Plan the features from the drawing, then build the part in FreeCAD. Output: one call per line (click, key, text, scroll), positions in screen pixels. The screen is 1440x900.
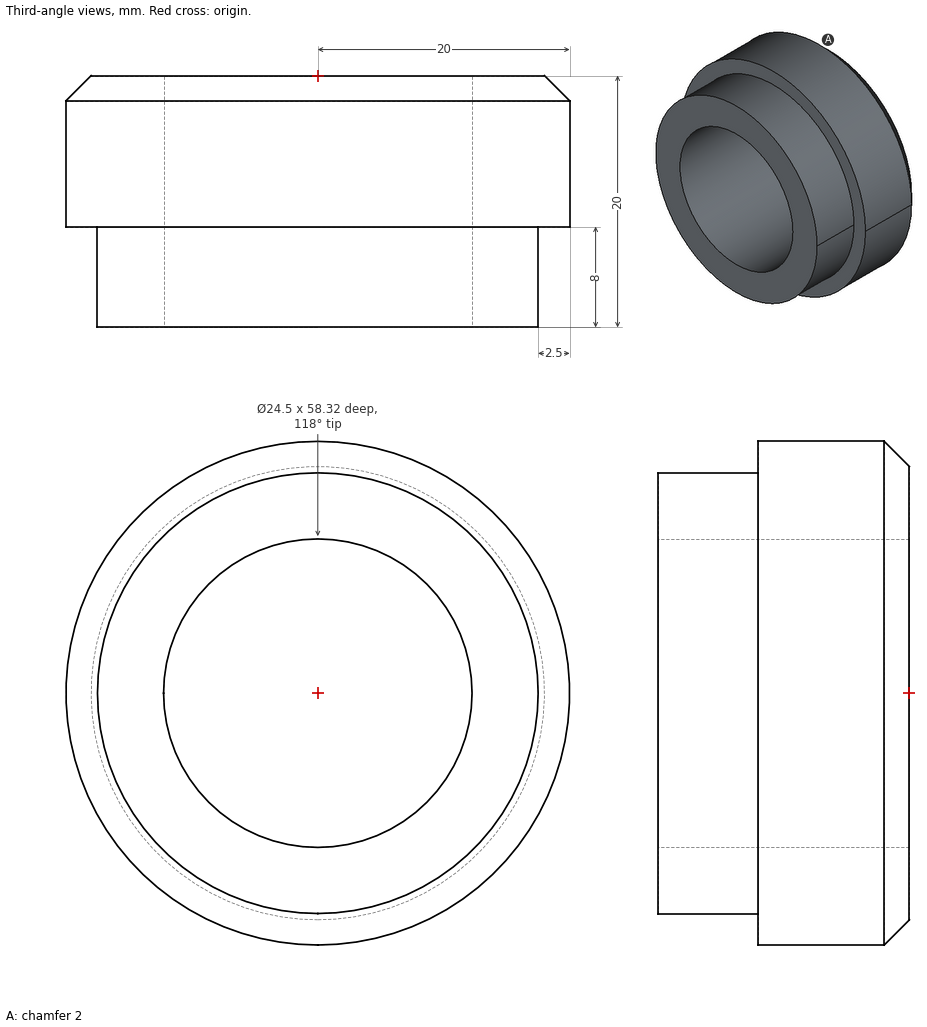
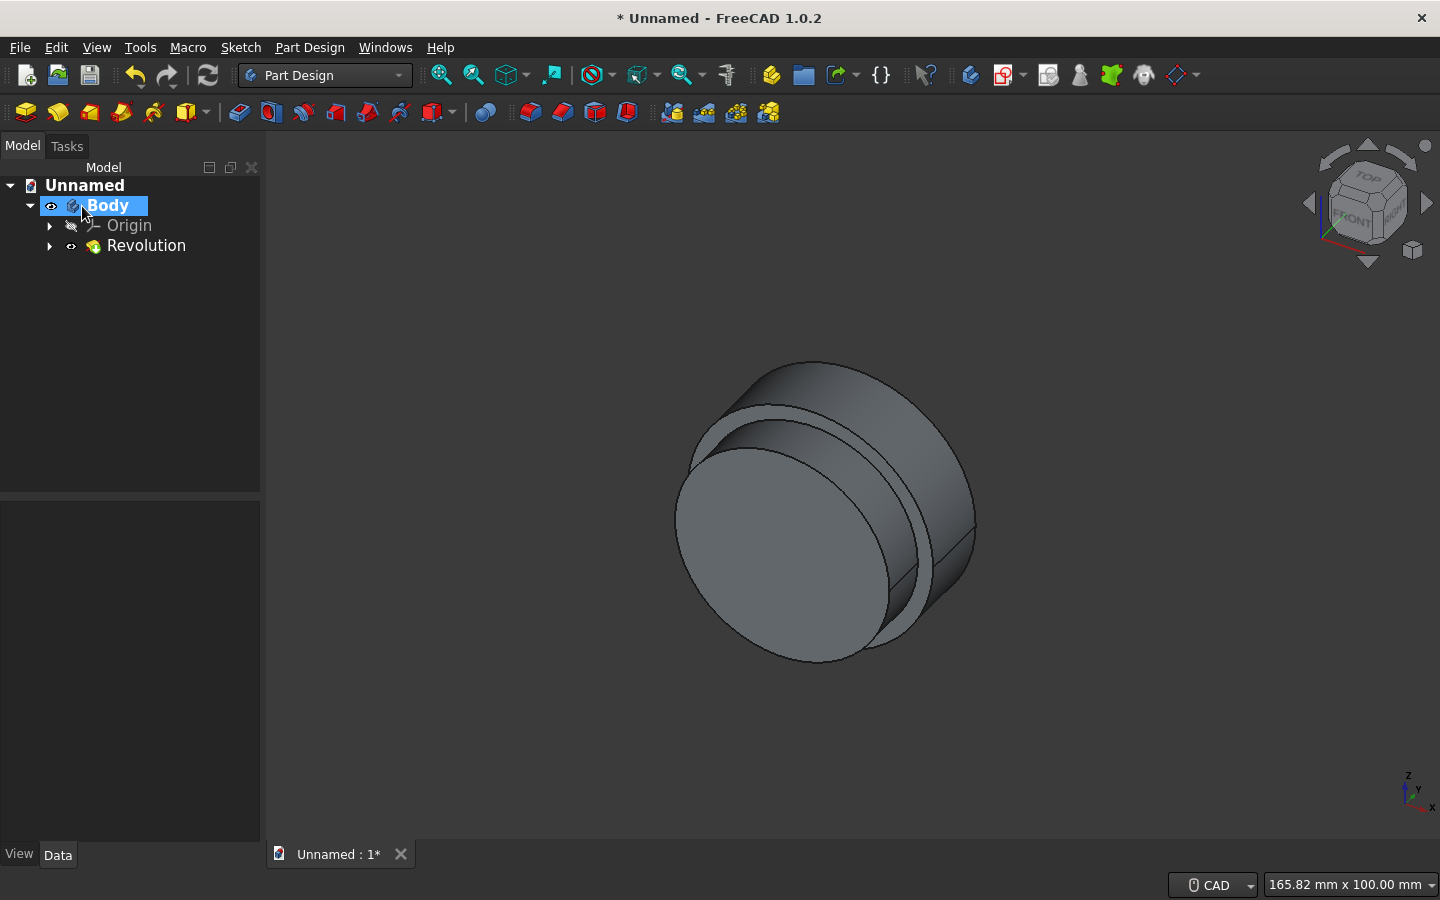
key(4)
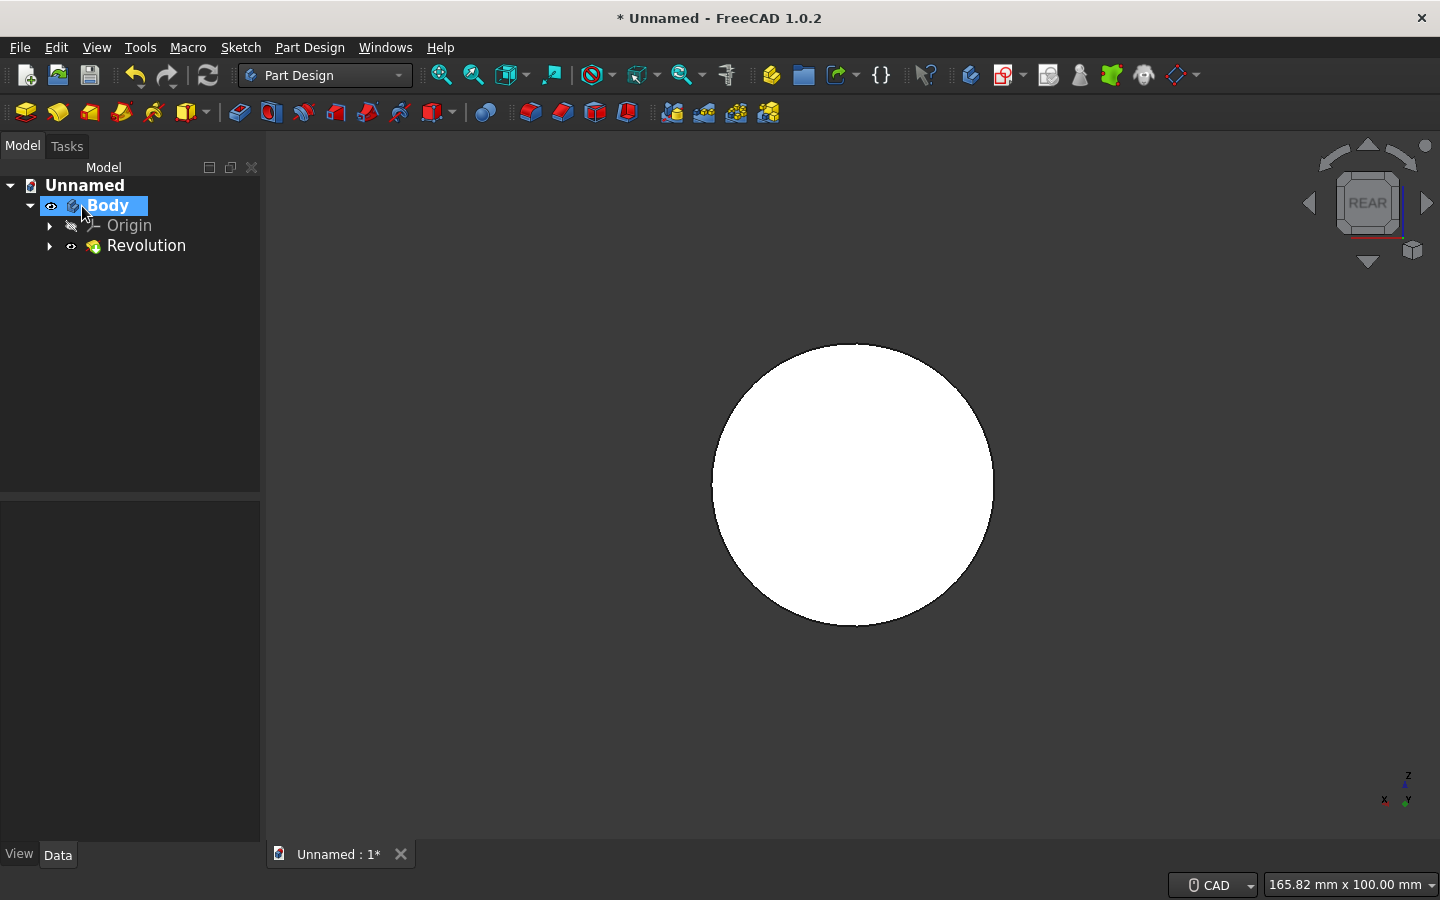
click(442, 76)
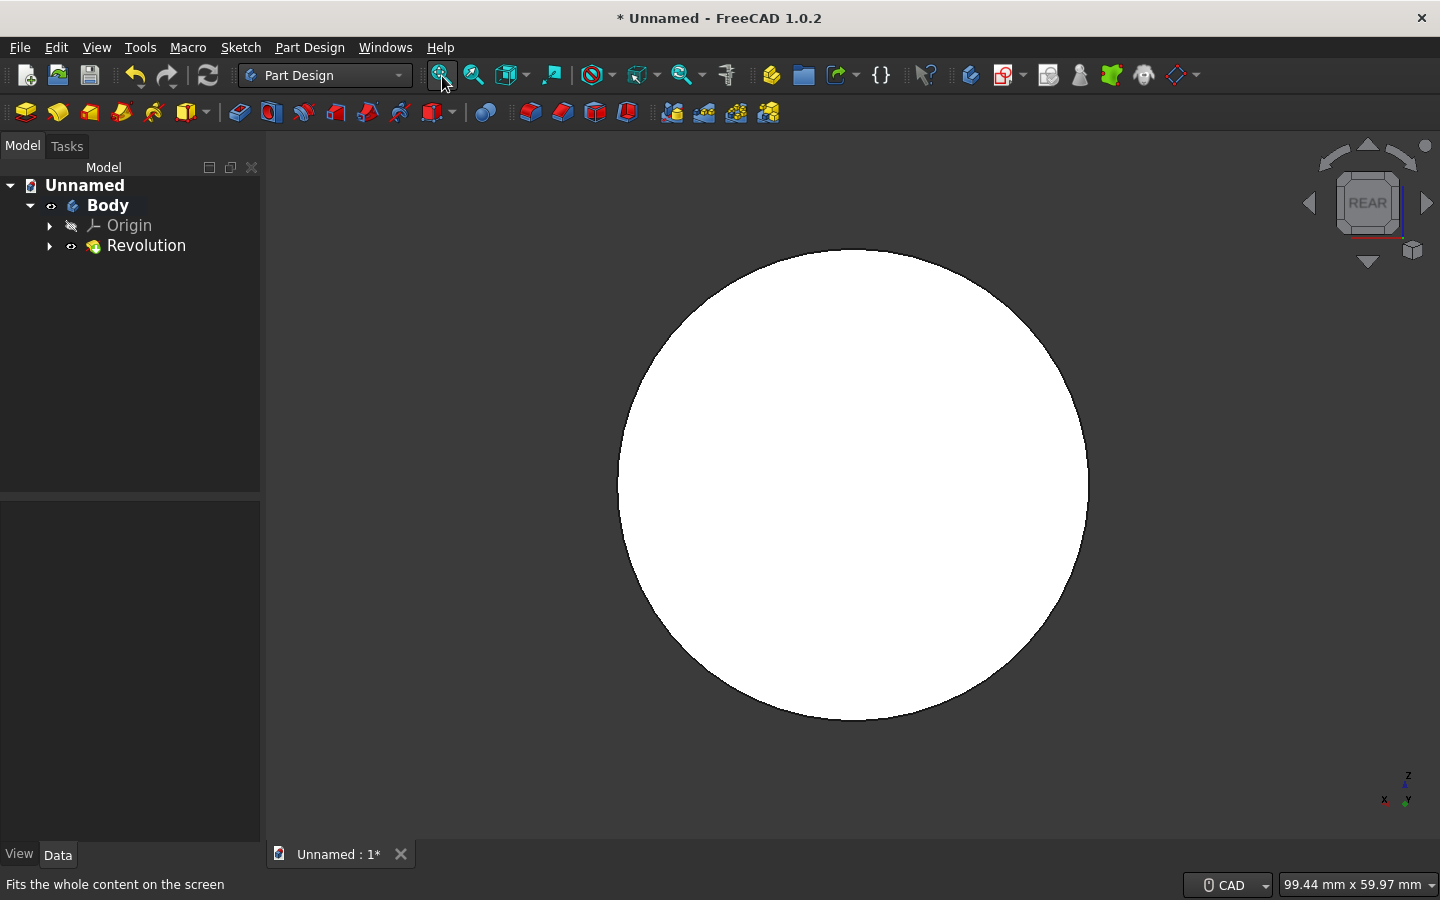
click(853, 484)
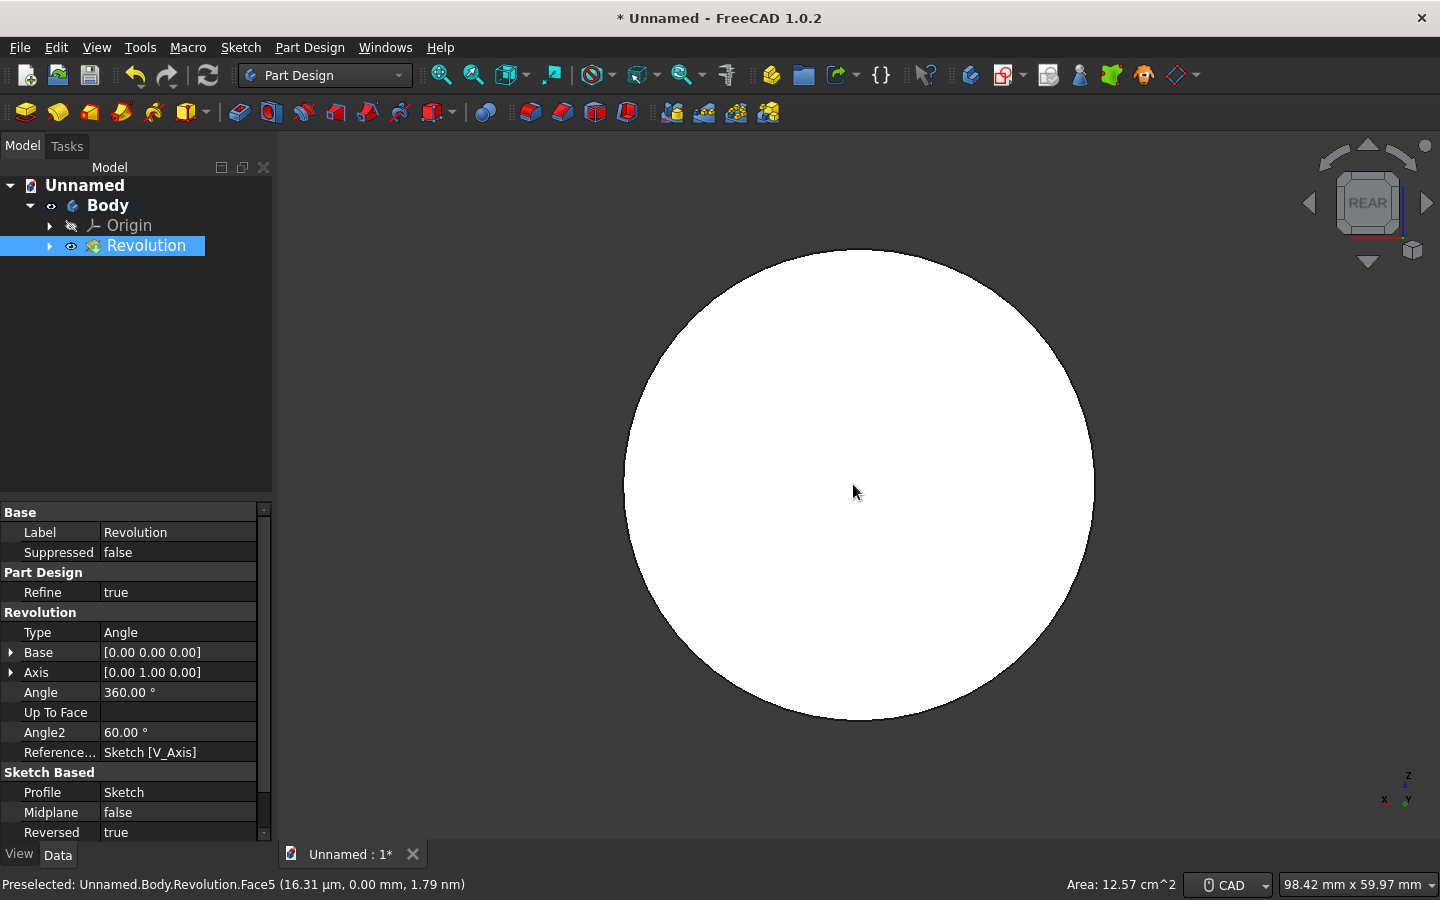
click(1004, 76)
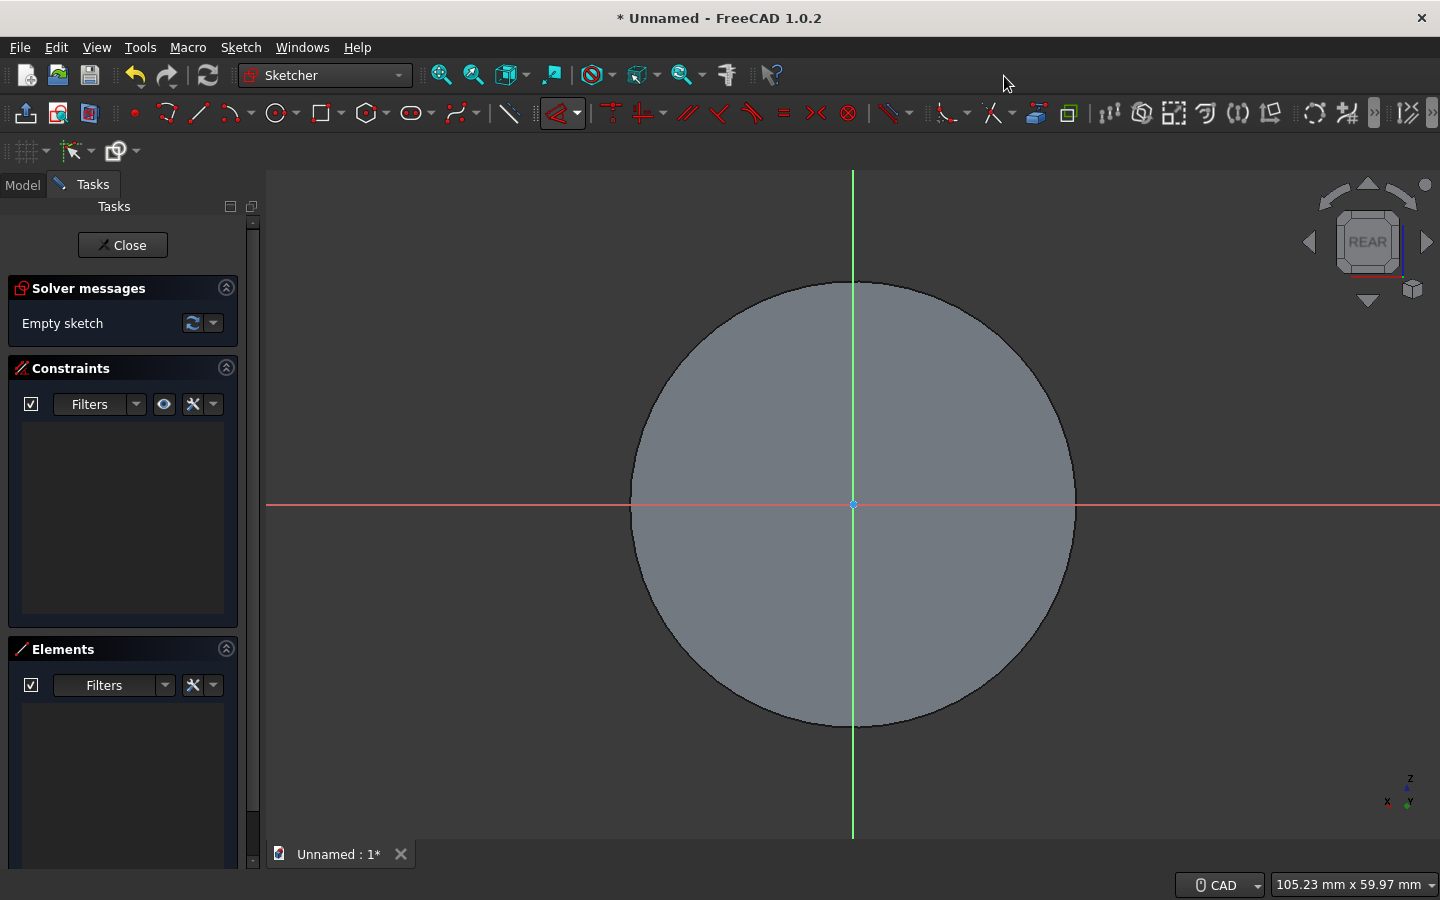
scroll(993, 505, up, 2)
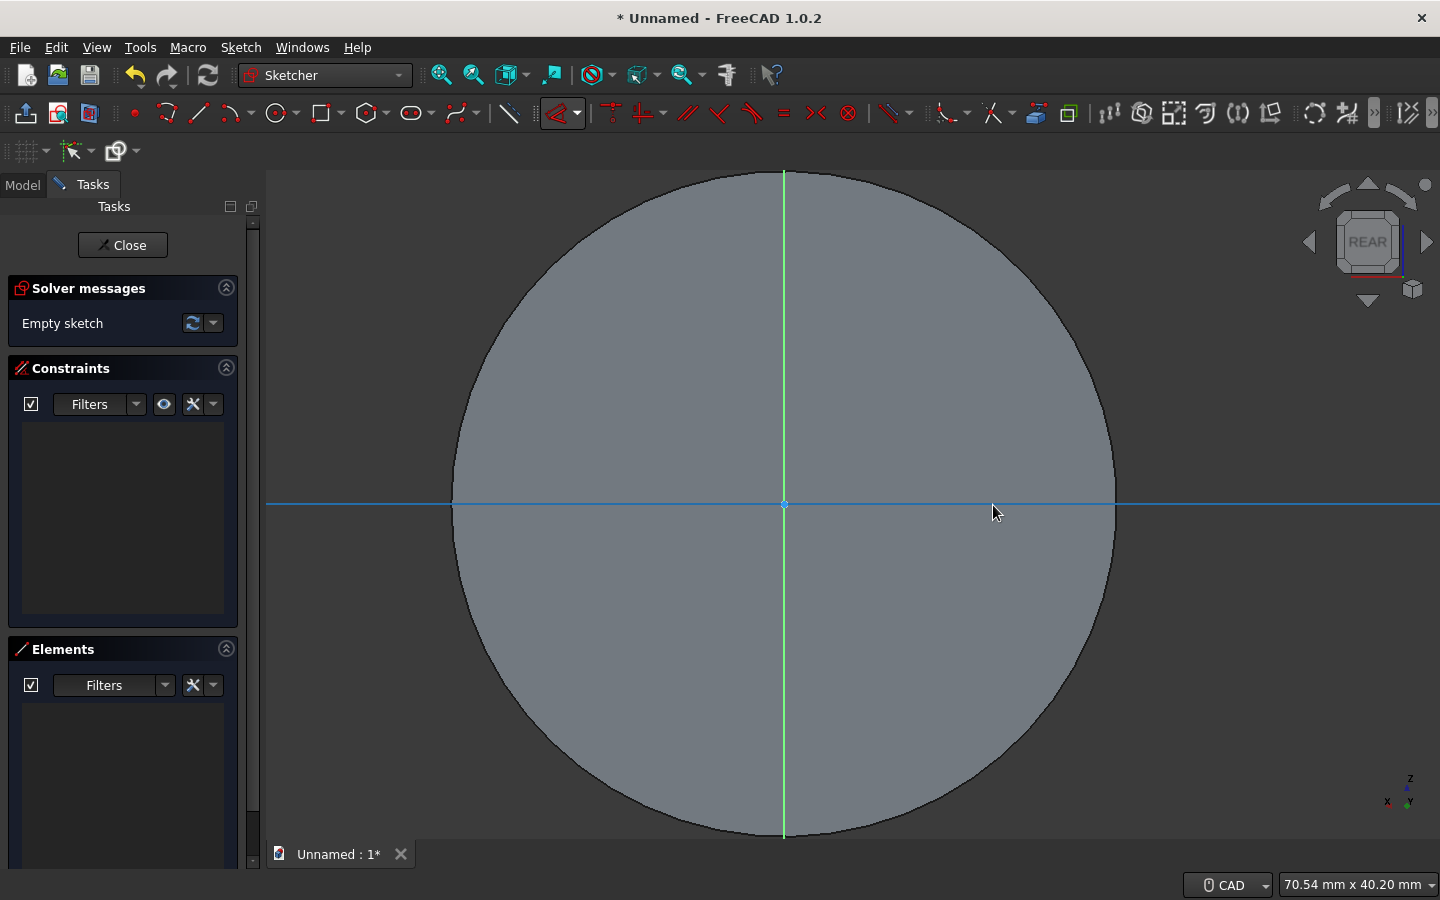
click(276, 114)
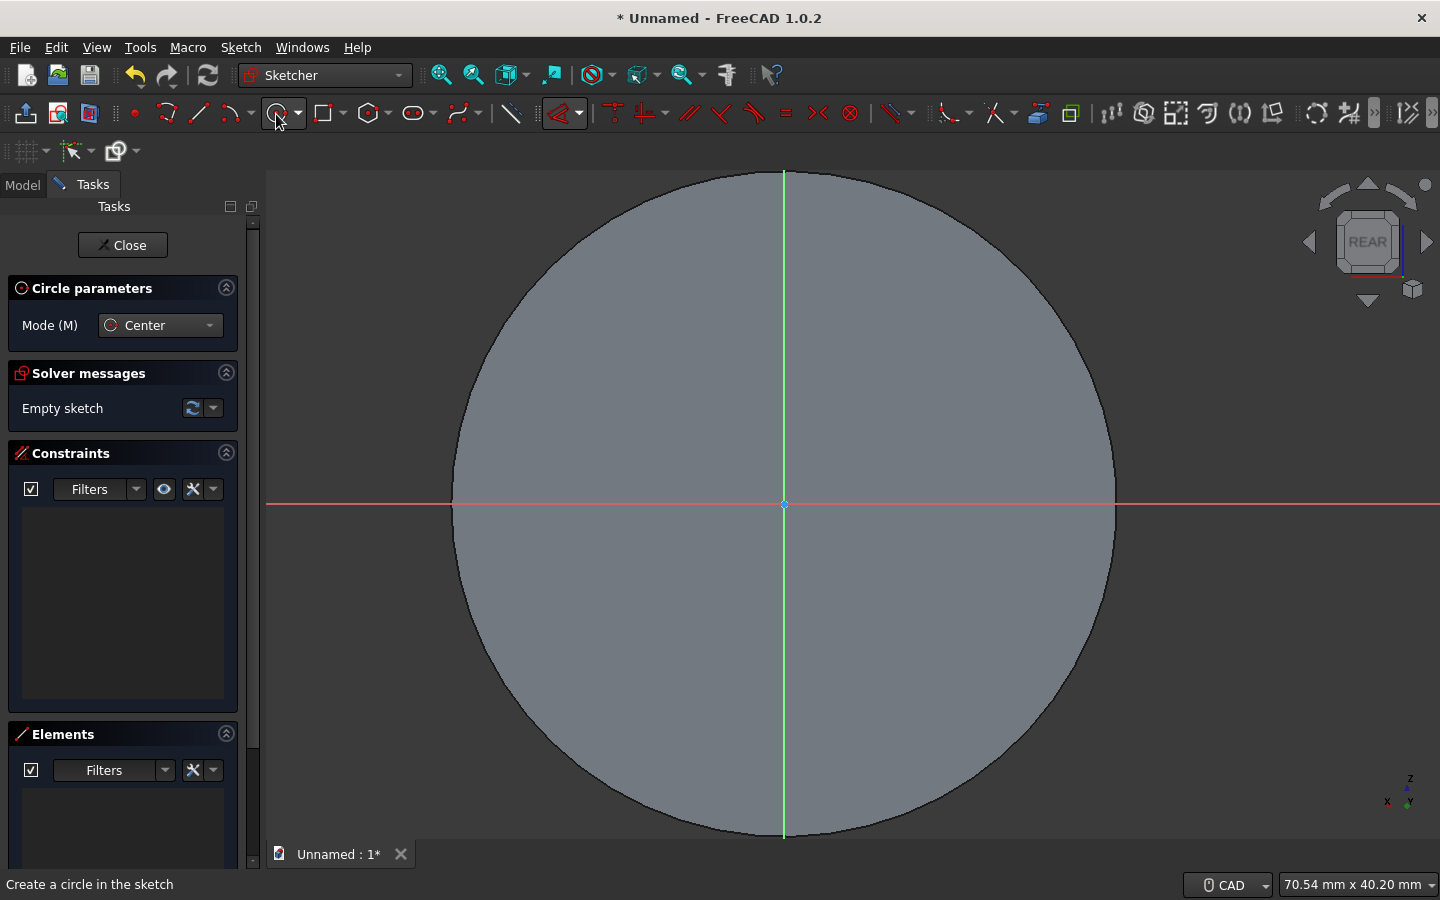
click(784, 504)
move(928, 360)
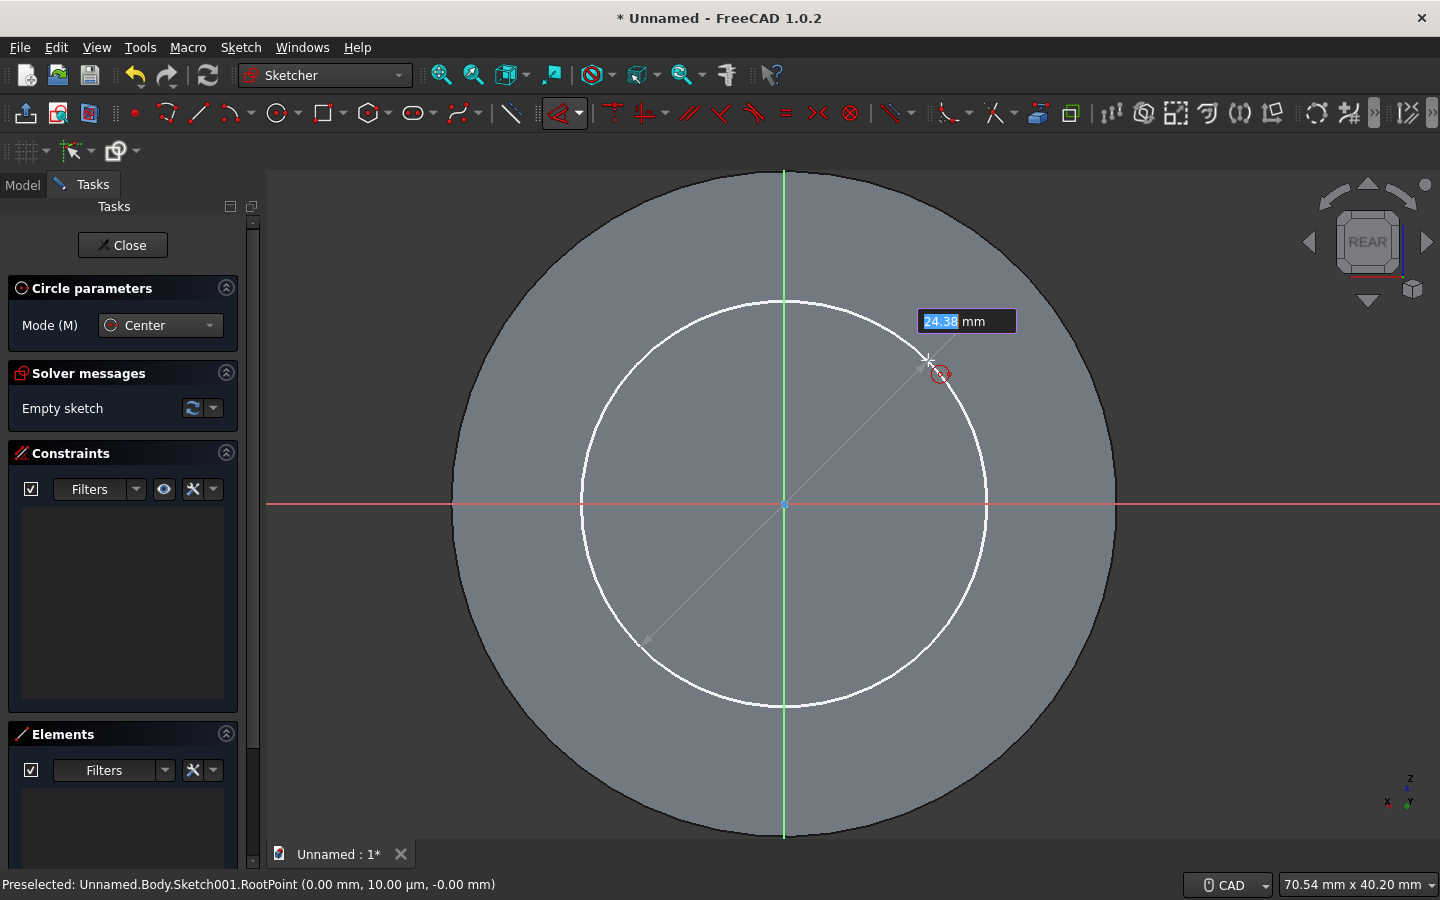
text(24.5)
key(Return)
key(Escape)